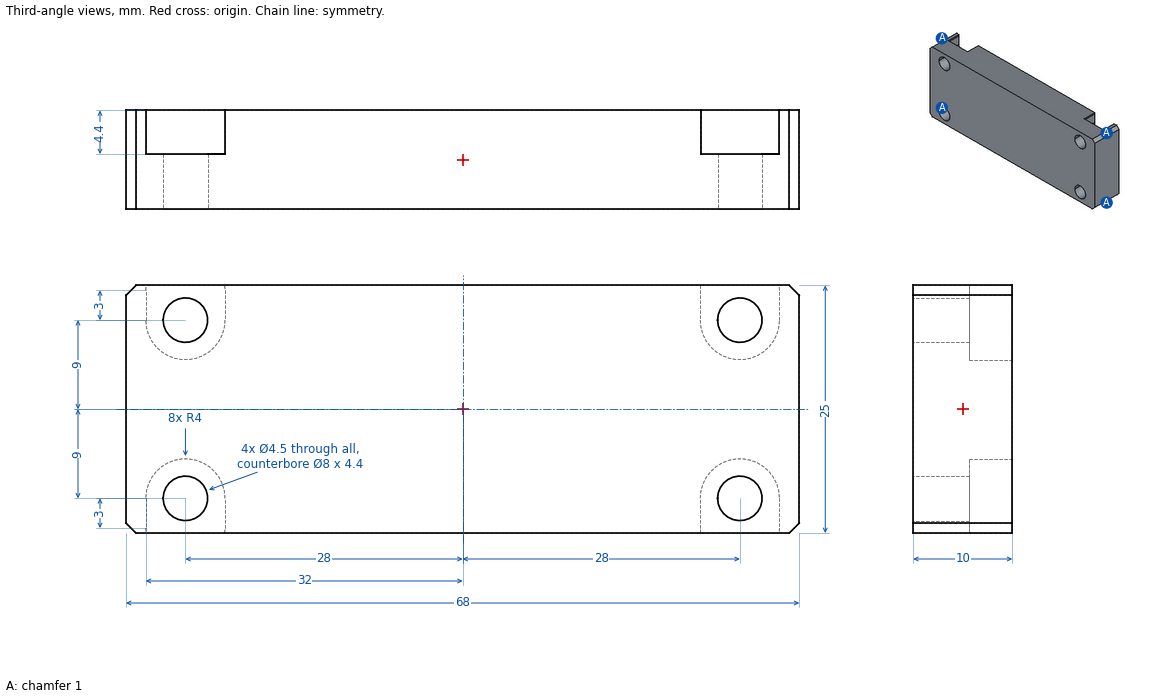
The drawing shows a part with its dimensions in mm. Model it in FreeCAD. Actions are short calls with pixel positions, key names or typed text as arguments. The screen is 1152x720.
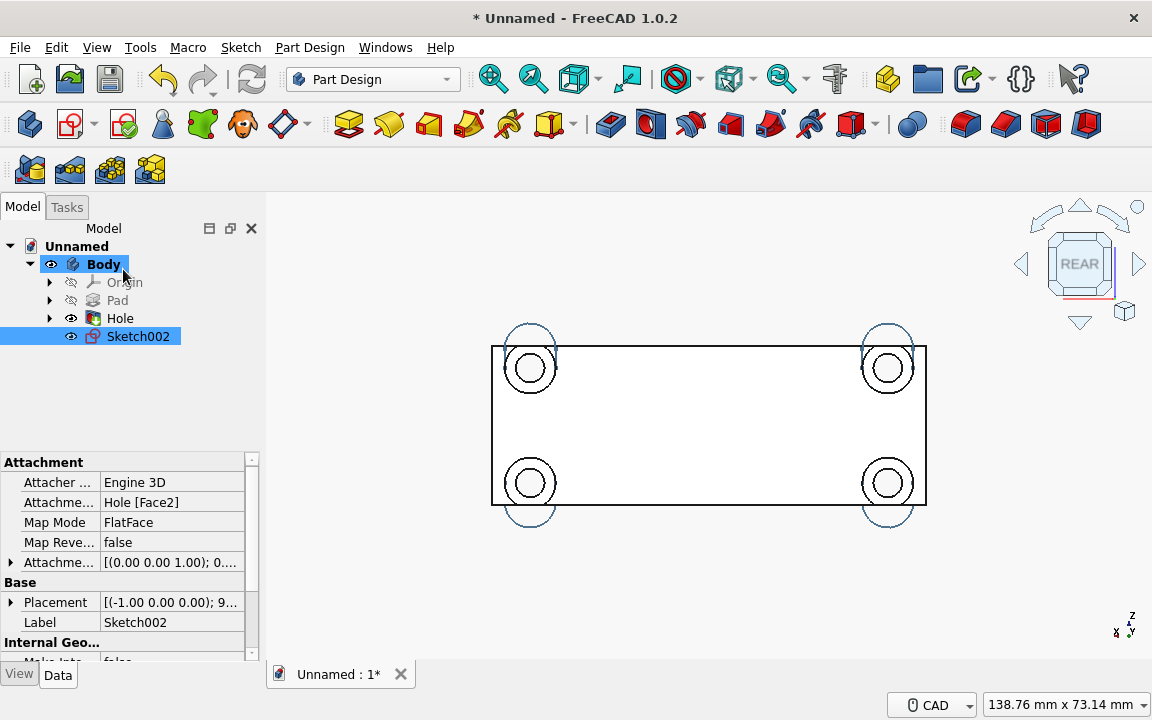
click(612, 124)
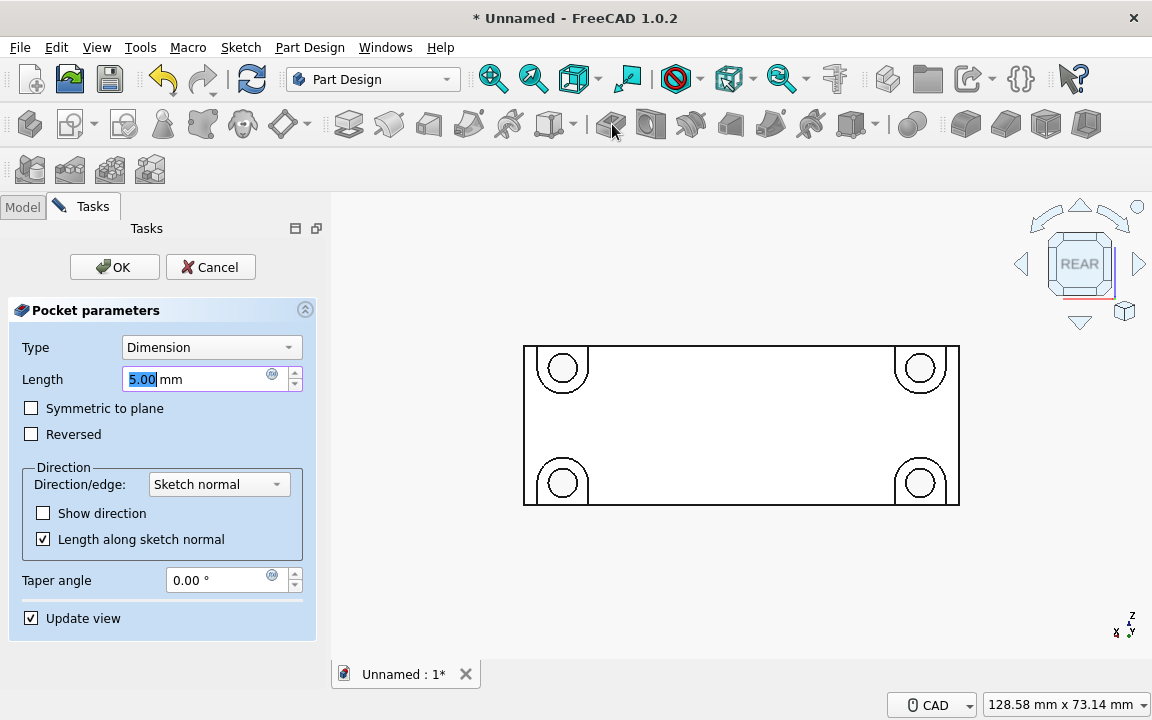
text(4.4)
key(Tab)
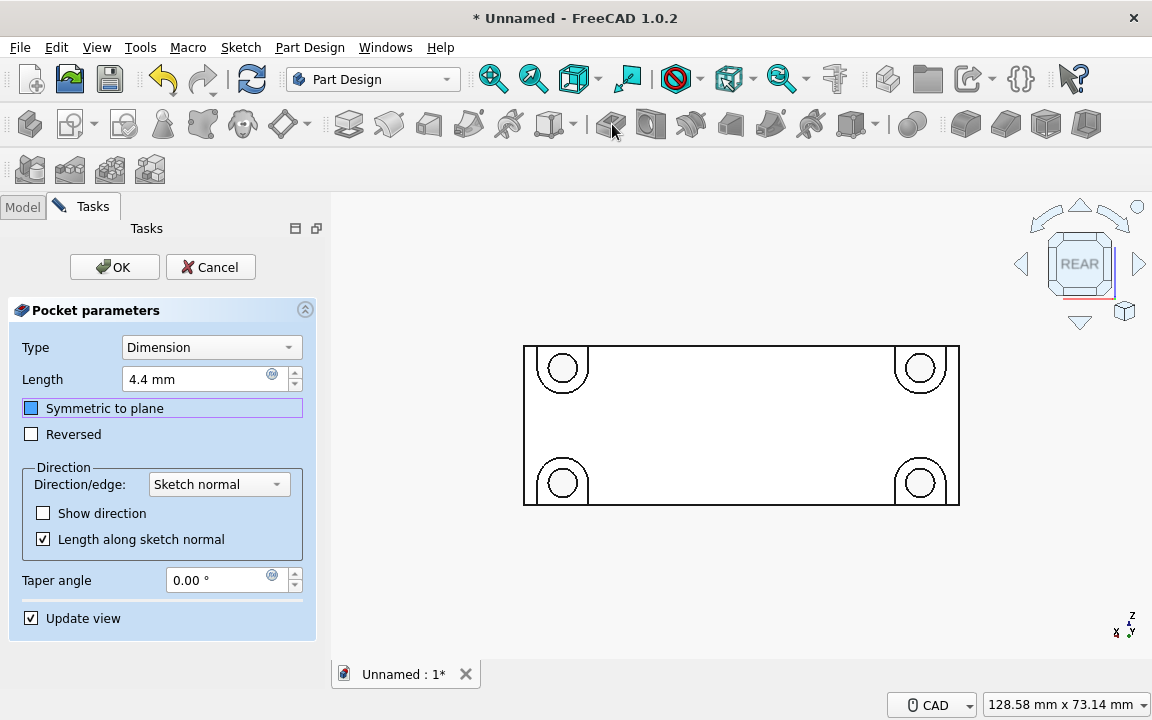
click(115, 267)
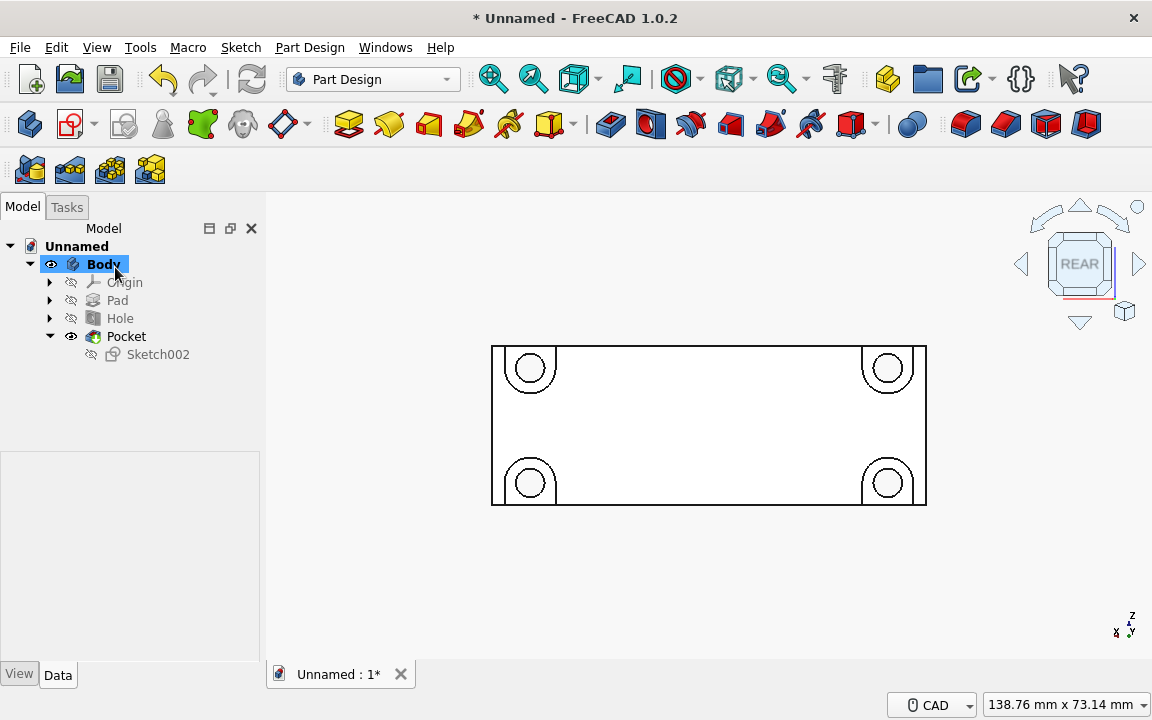
key(0)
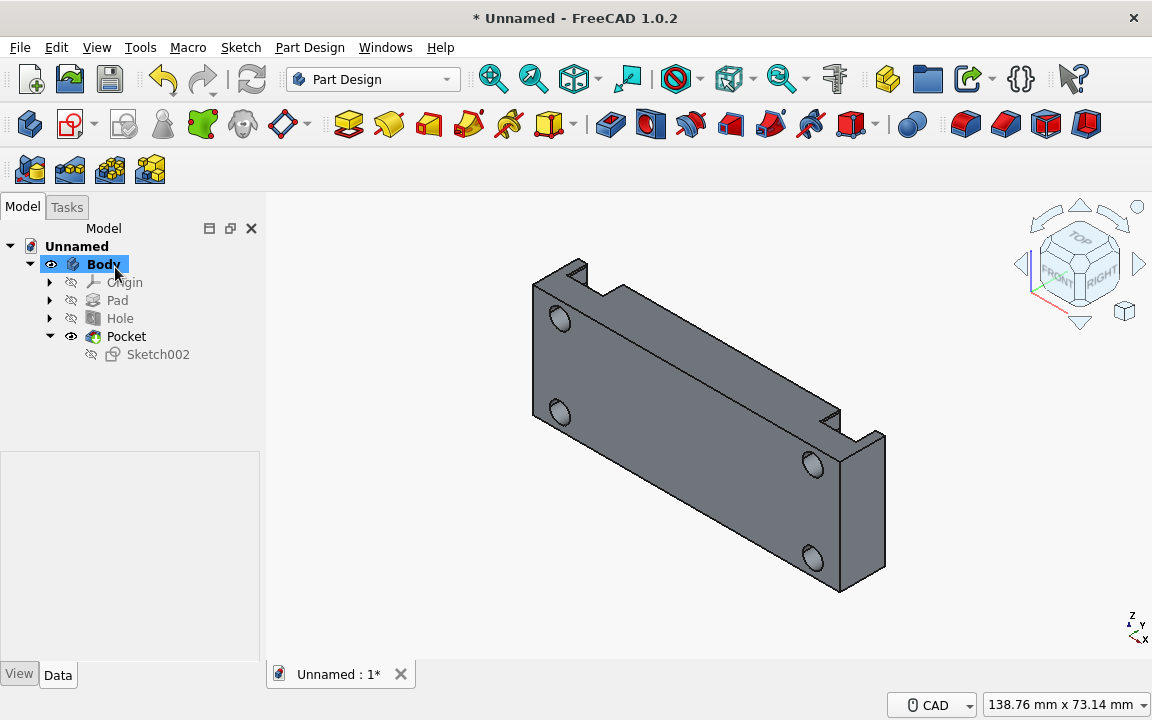
click(863, 448)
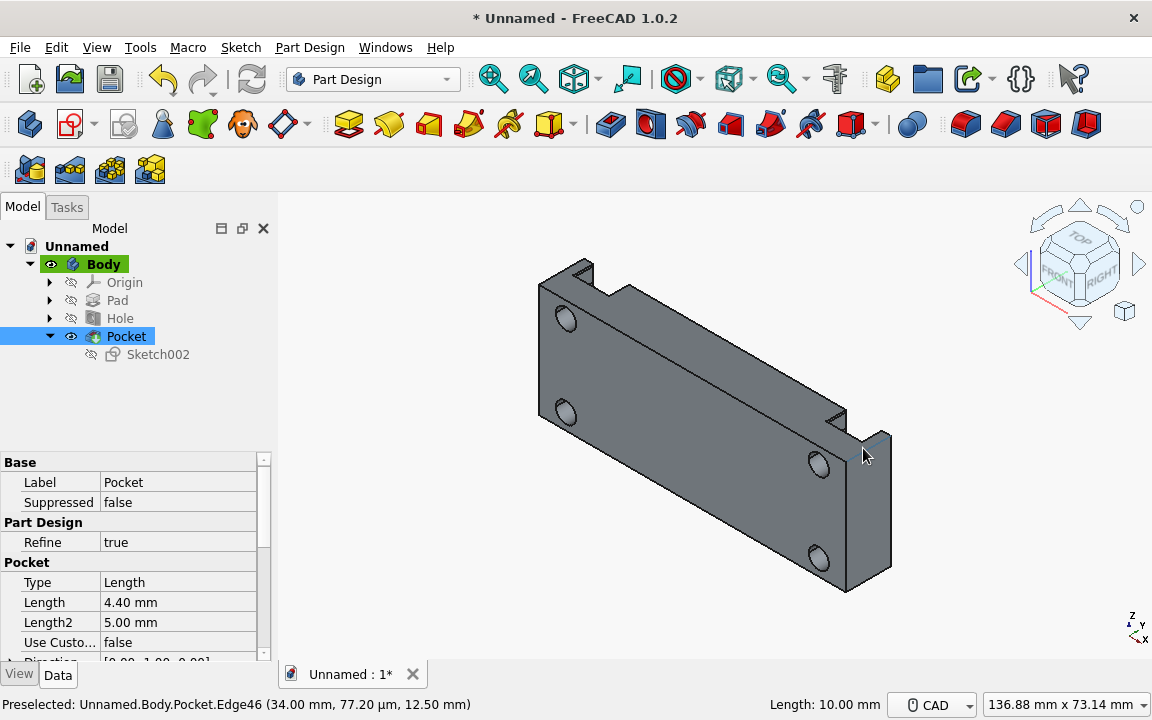
key(2)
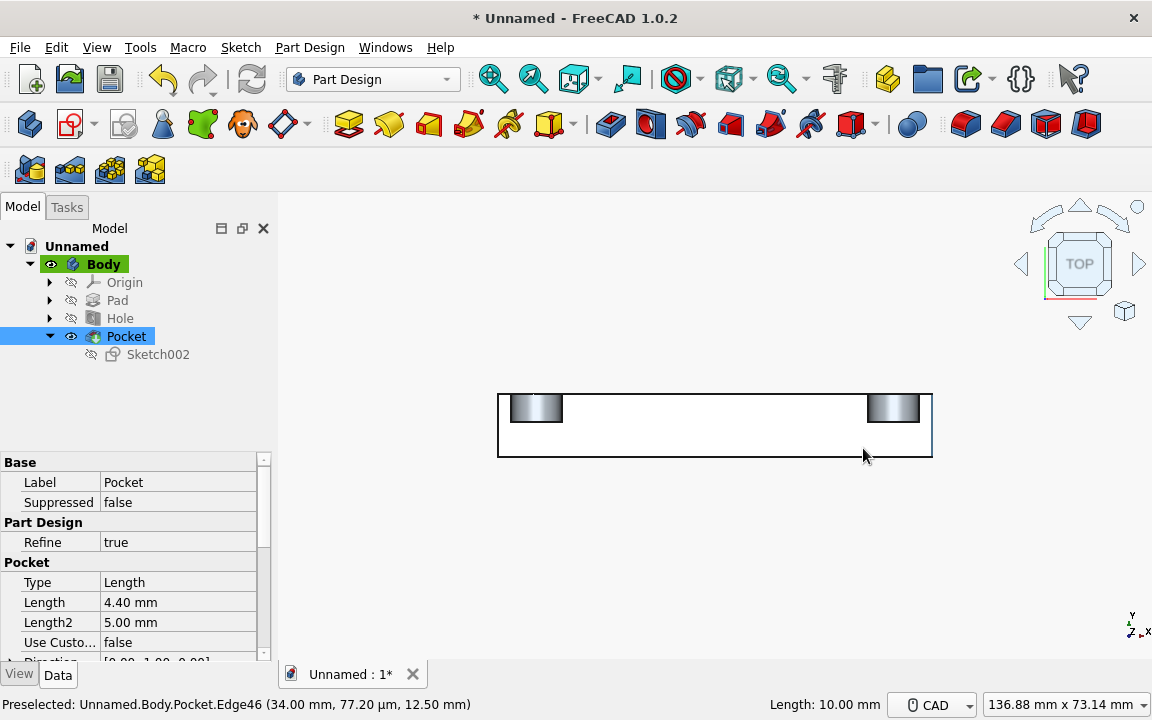
click(498, 424, ctrl)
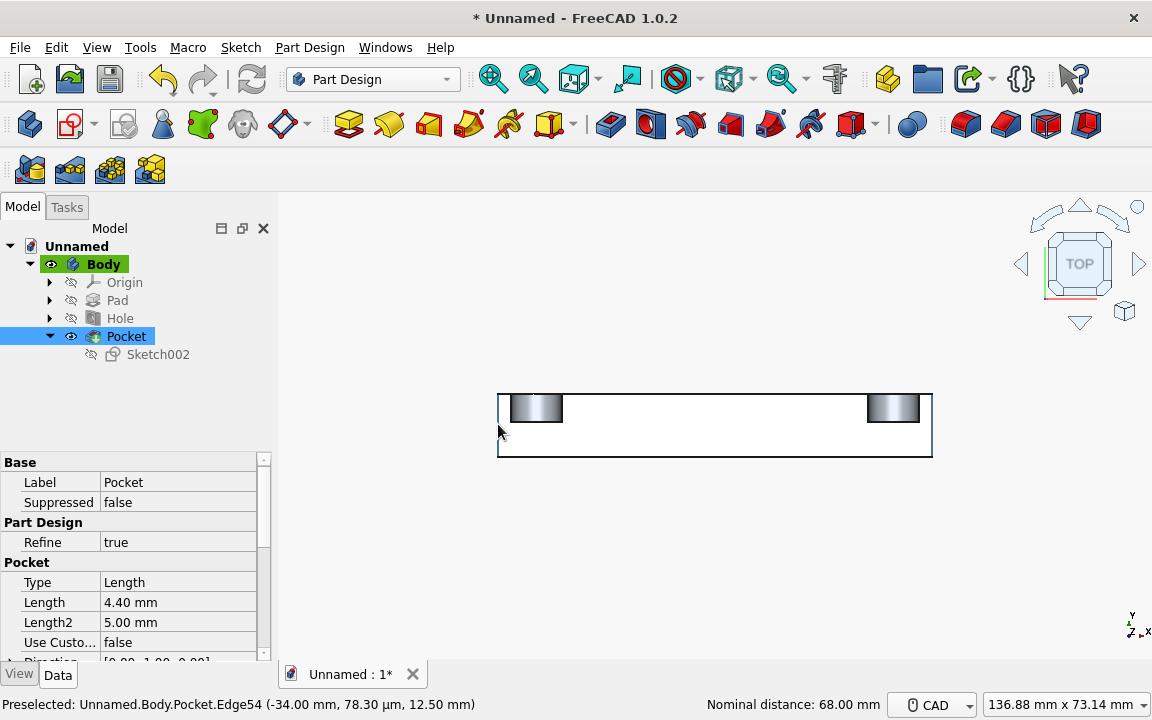
key(1)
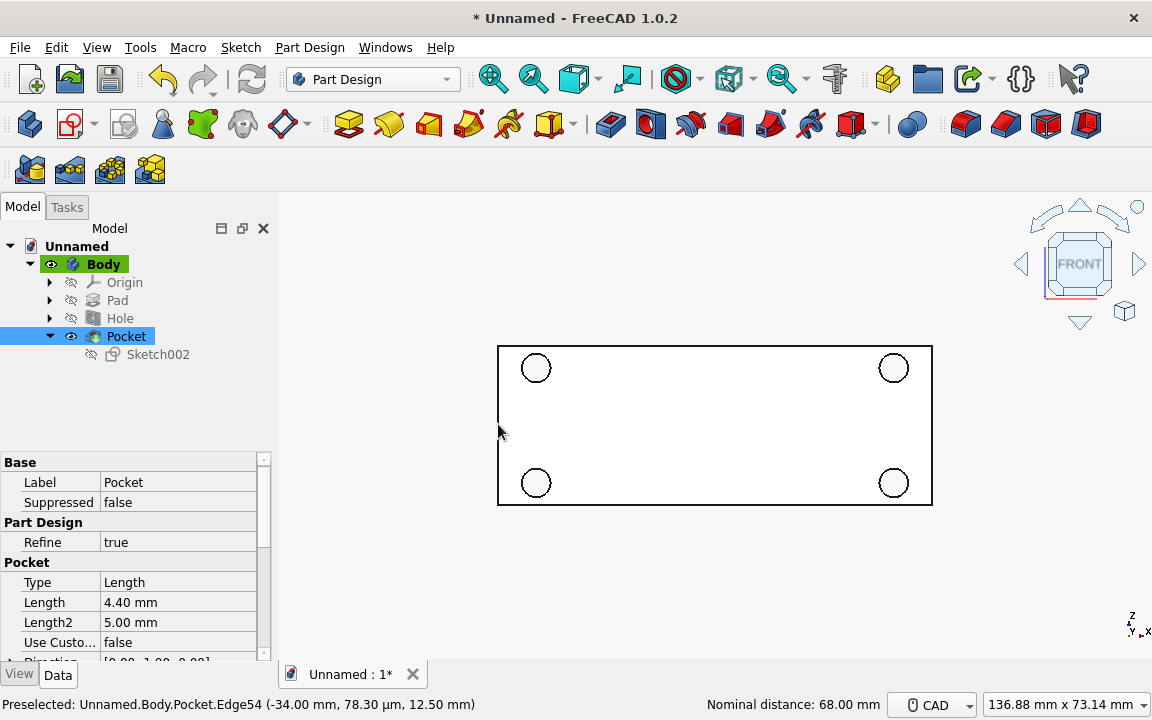
key(3)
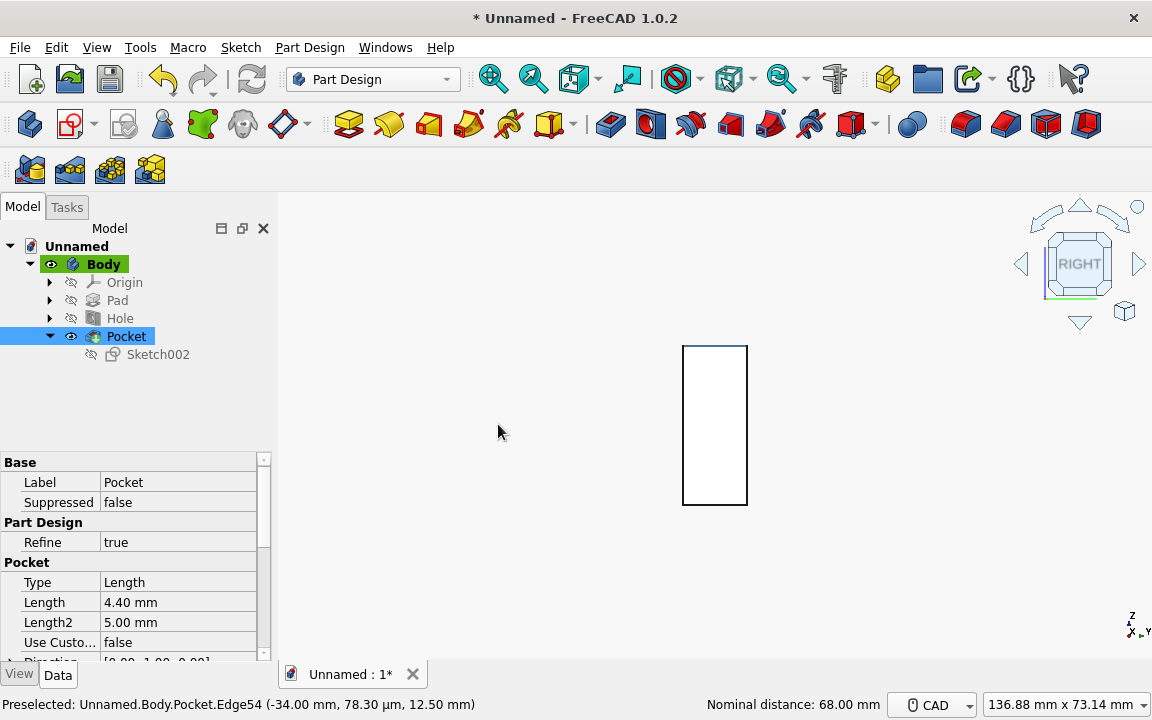
click(494, 80)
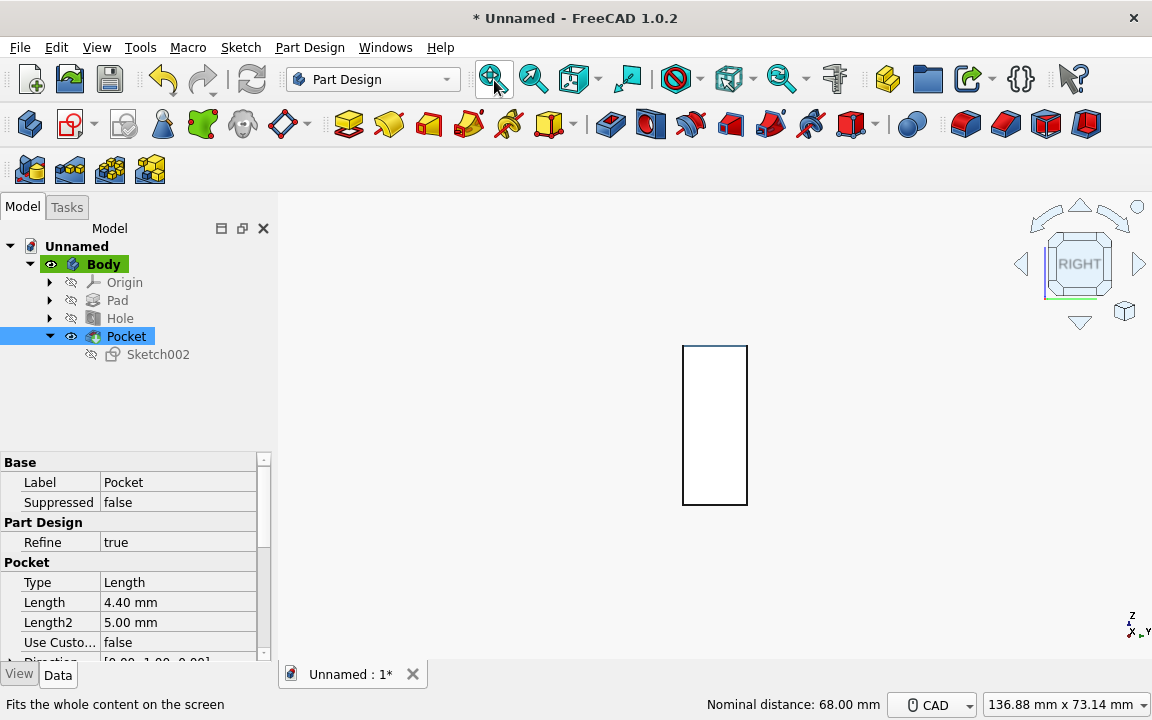
click(715, 504, ctrl)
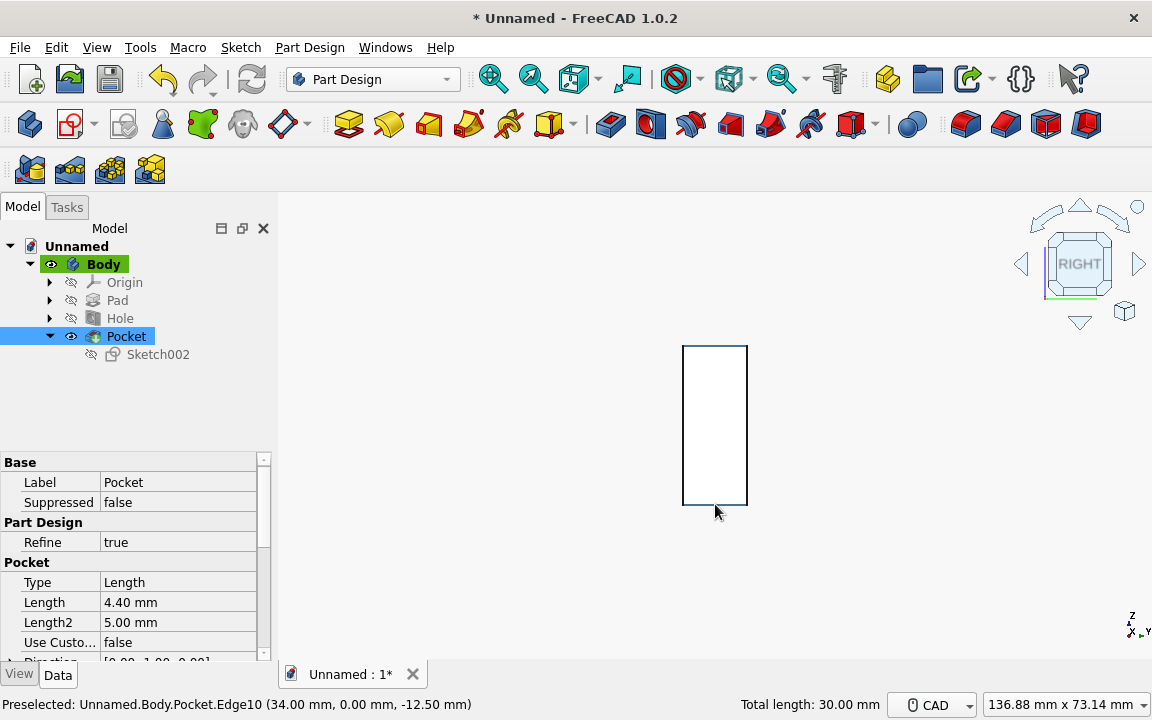
key(5)